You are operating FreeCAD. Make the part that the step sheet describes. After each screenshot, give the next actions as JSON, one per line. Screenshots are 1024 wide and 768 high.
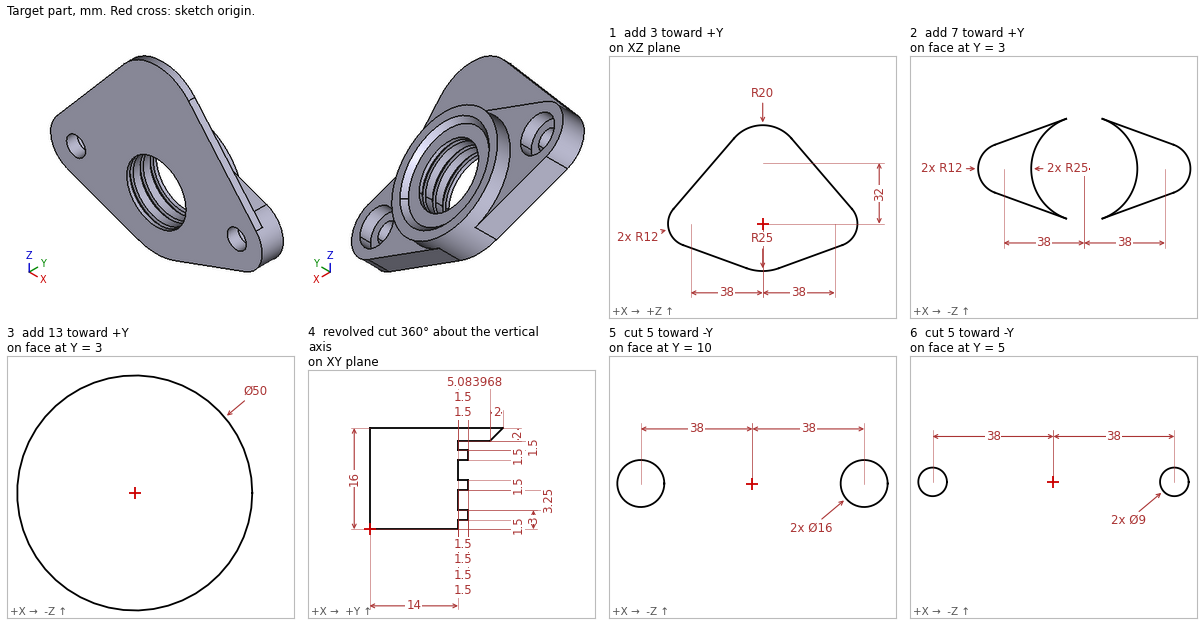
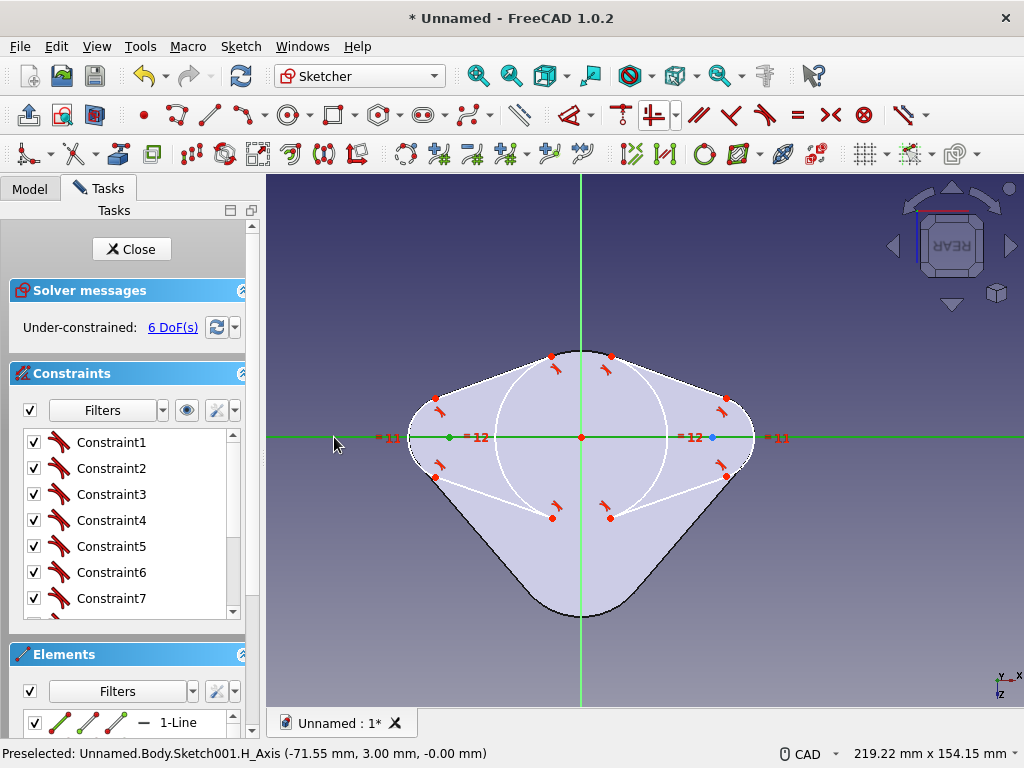
{"action": "left_click", "coordinate": [621, 116]}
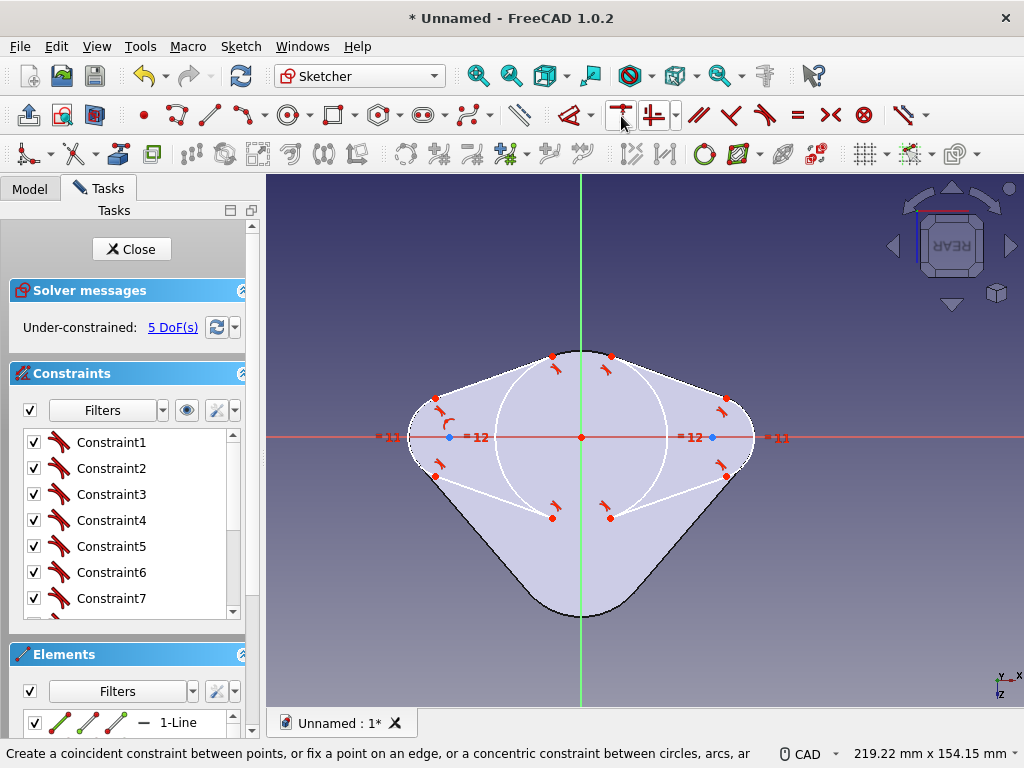
{"action": "left_click", "coordinate": [713, 438]}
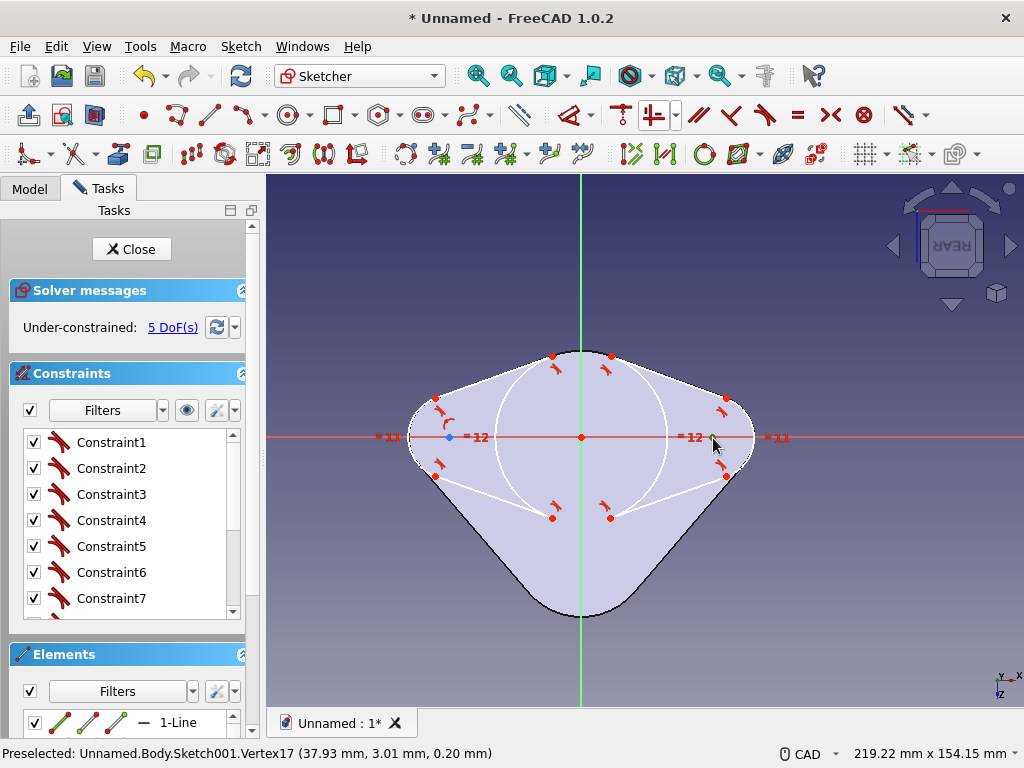
{"action": "left_click", "coordinate": [334, 437]}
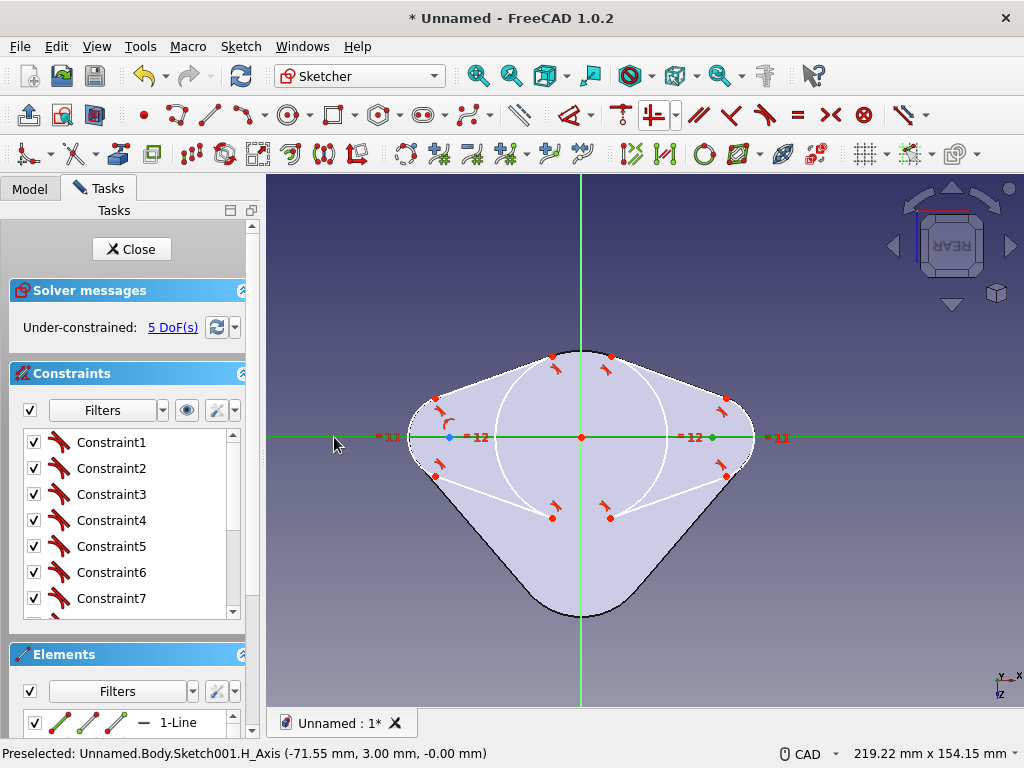
{"action": "left_click", "coordinate": [621, 116]}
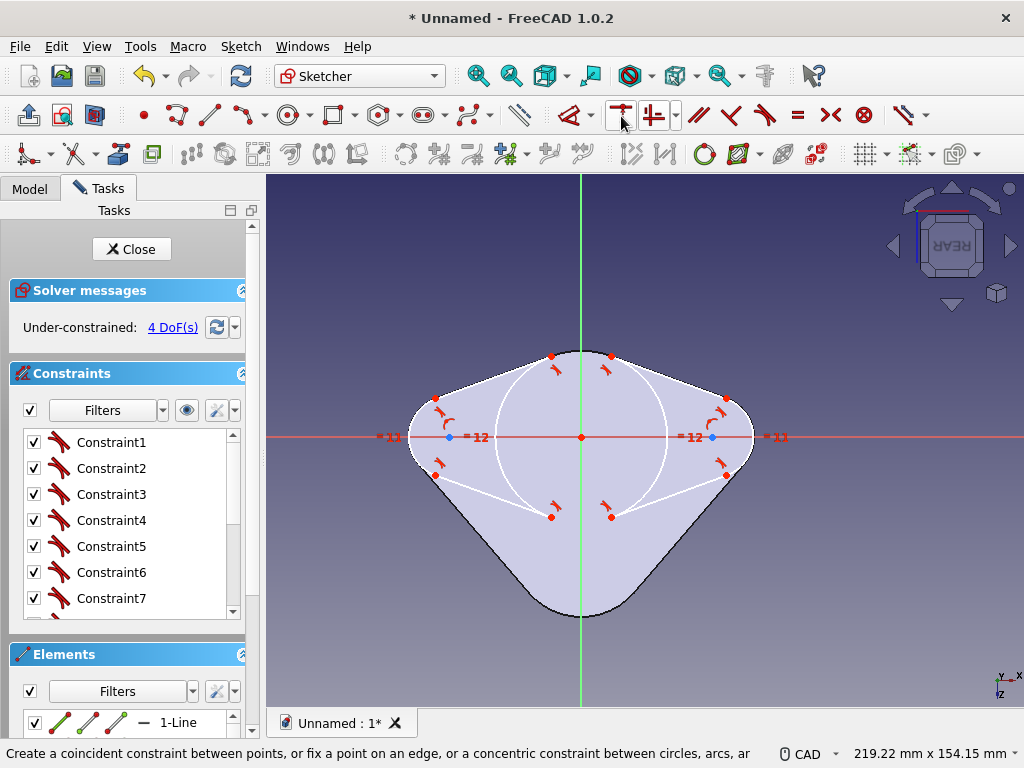
{"action": "left_click", "coordinate": [568, 116]}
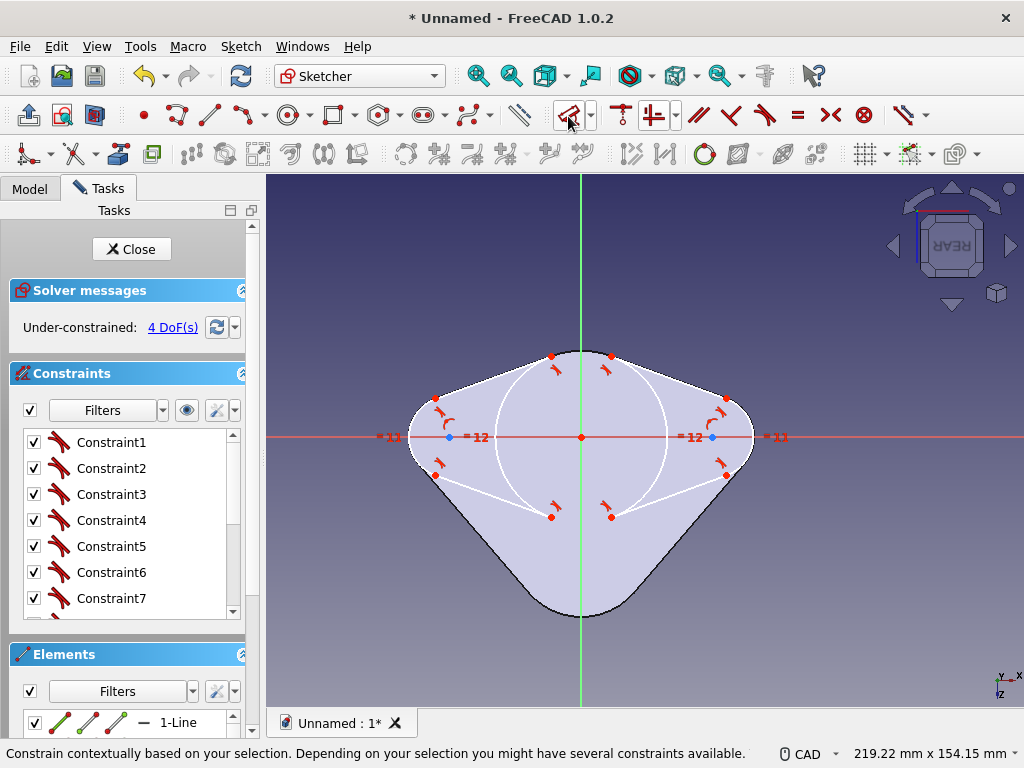
{"action": "left_click", "coordinate": [505, 397]}
{"action": "left_click", "coordinate": [516, 339]}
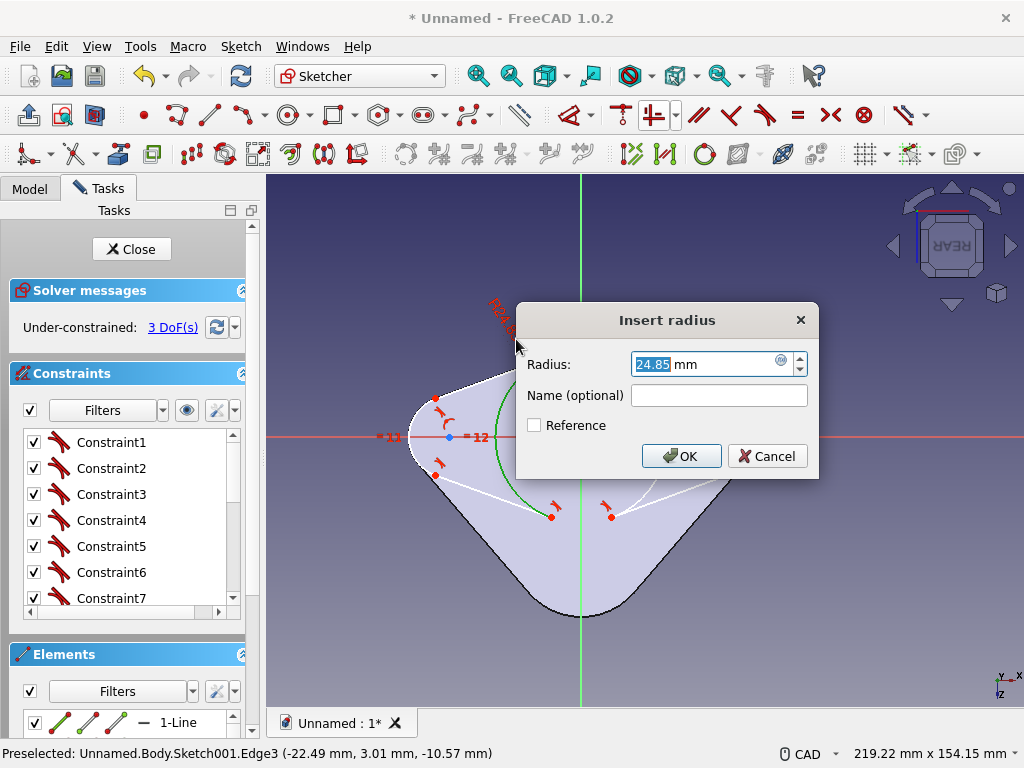
{"action": "type", "text": "25"}
{"action": "key", "text": "Return"}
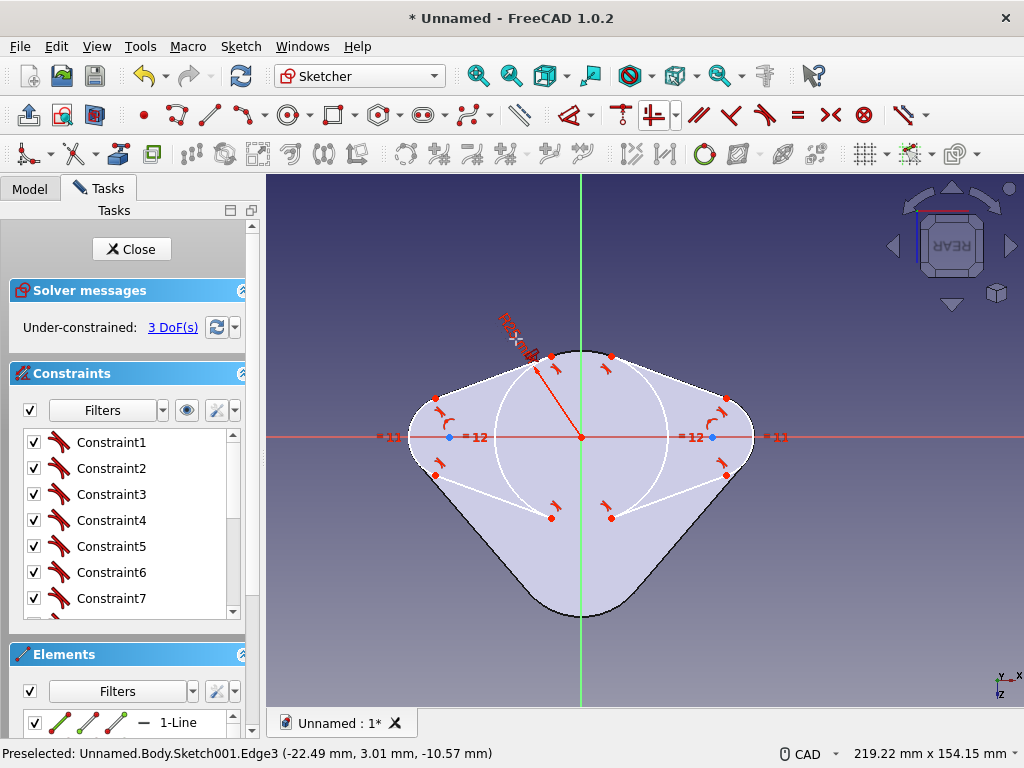
{"action": "left_click", "coordinate": [414, 418]}
{"action": "left_click", "coordinate": [386, 403]}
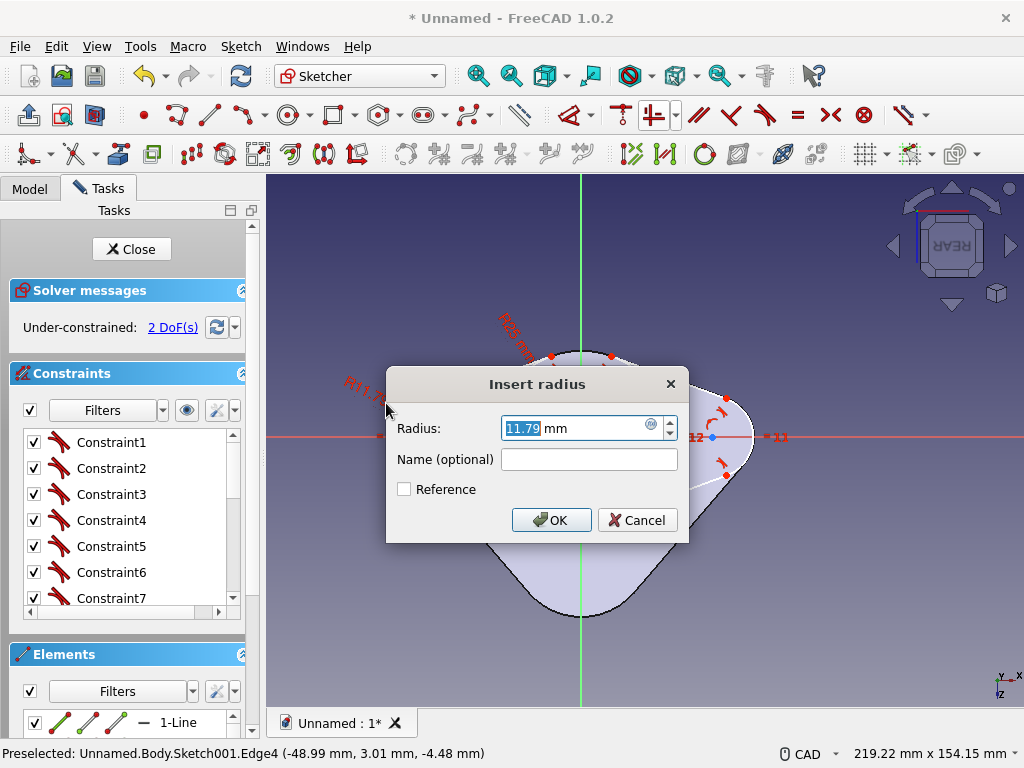
{"action": "type", "text": "12"}
{"action": "key", "text": "Return"}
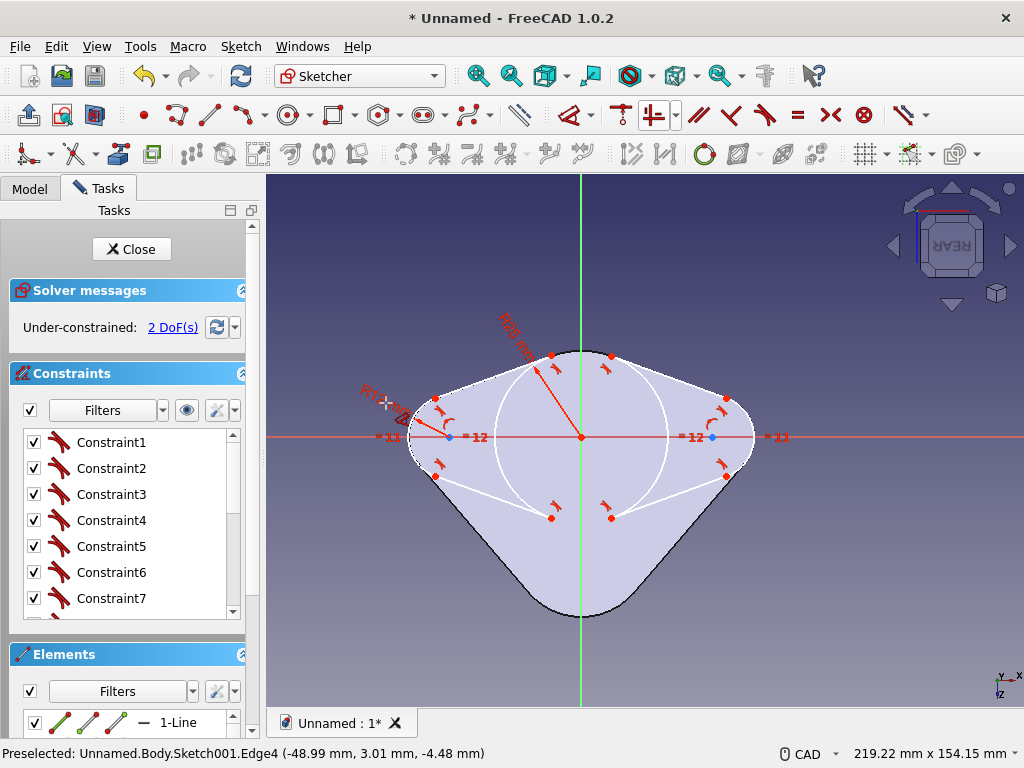
{"action": "left_click", "coordinate": [450, 437]}
{"action": "left_click", "coordinate": [485, 471]}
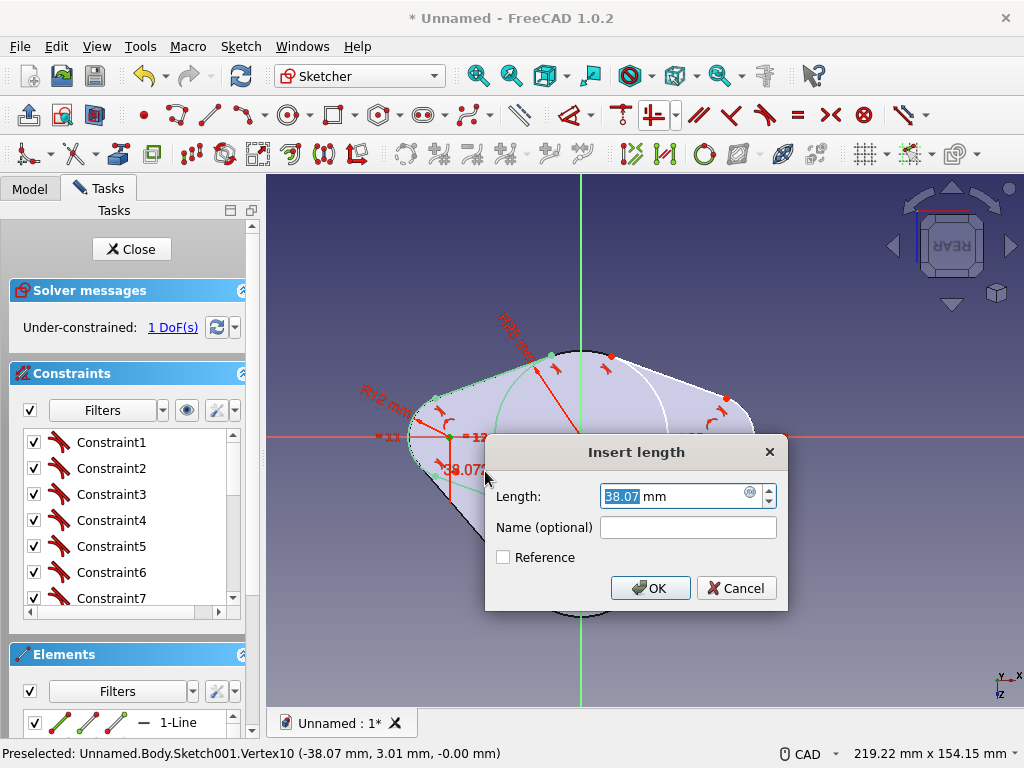
{"action": "type", "text": "38"}
{"action": "key", "text": "Return"}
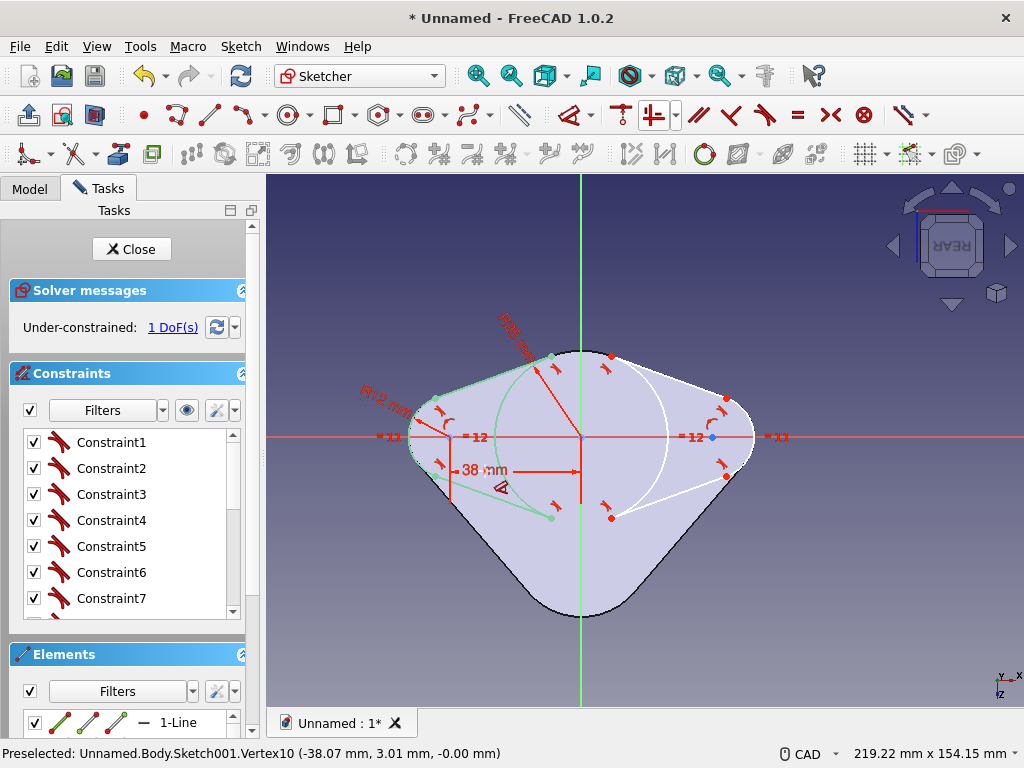
{"action": "left_click", "coordinate": [713, 437]}
{"action": "left_click", "coordinate": [617, 471]}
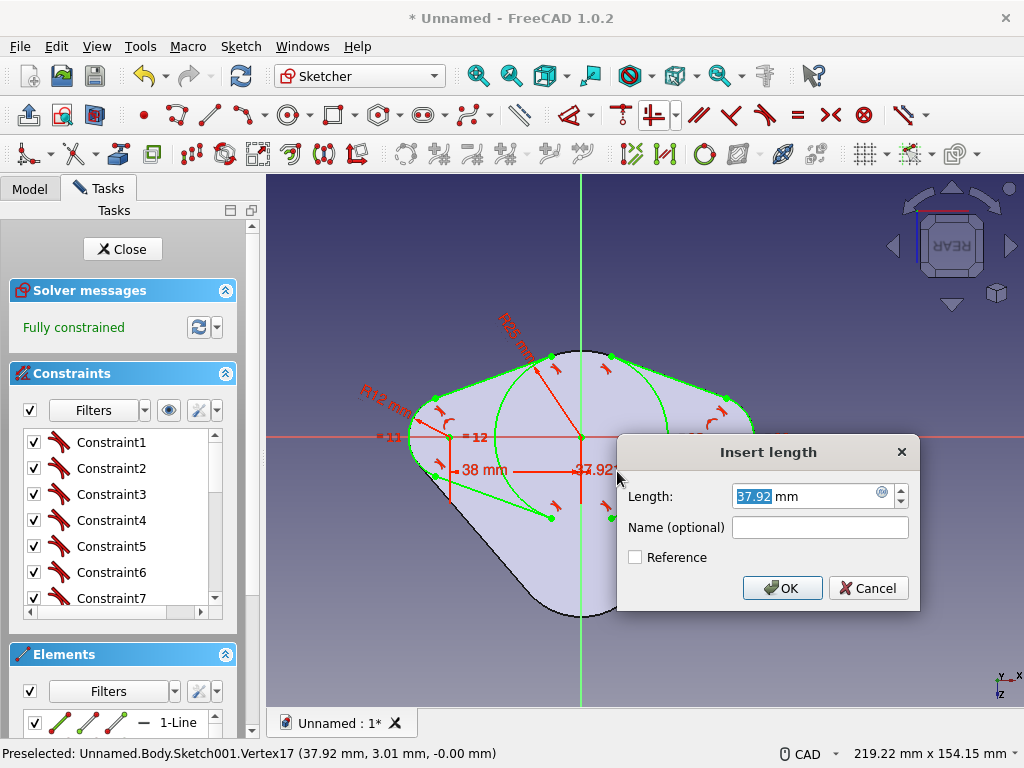
{"action": "type", "text": "38"}
{"action": "key", "text": "Return"}
{"action": "key", "text": "Escape"}